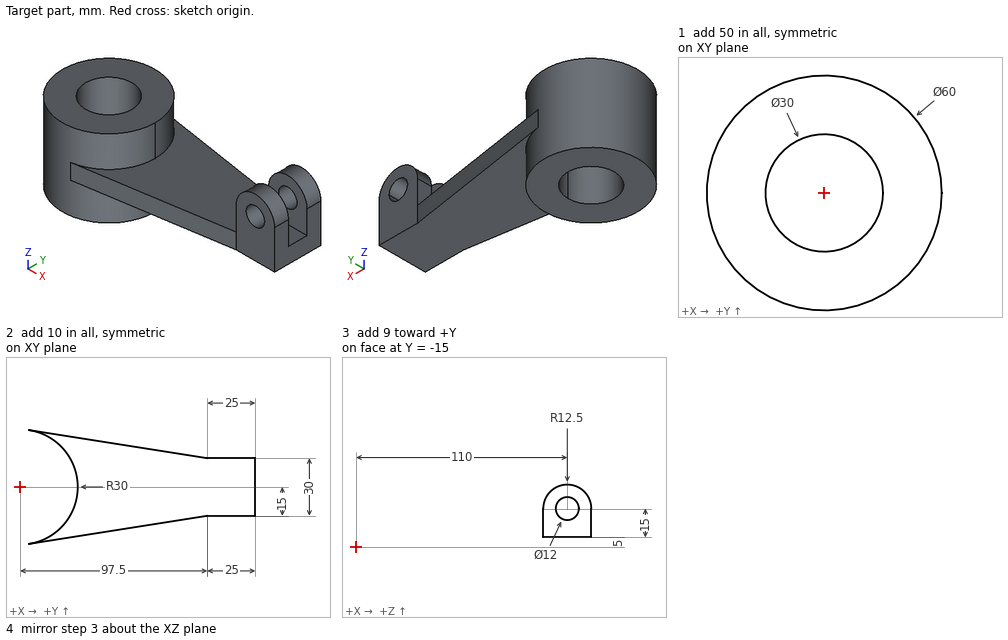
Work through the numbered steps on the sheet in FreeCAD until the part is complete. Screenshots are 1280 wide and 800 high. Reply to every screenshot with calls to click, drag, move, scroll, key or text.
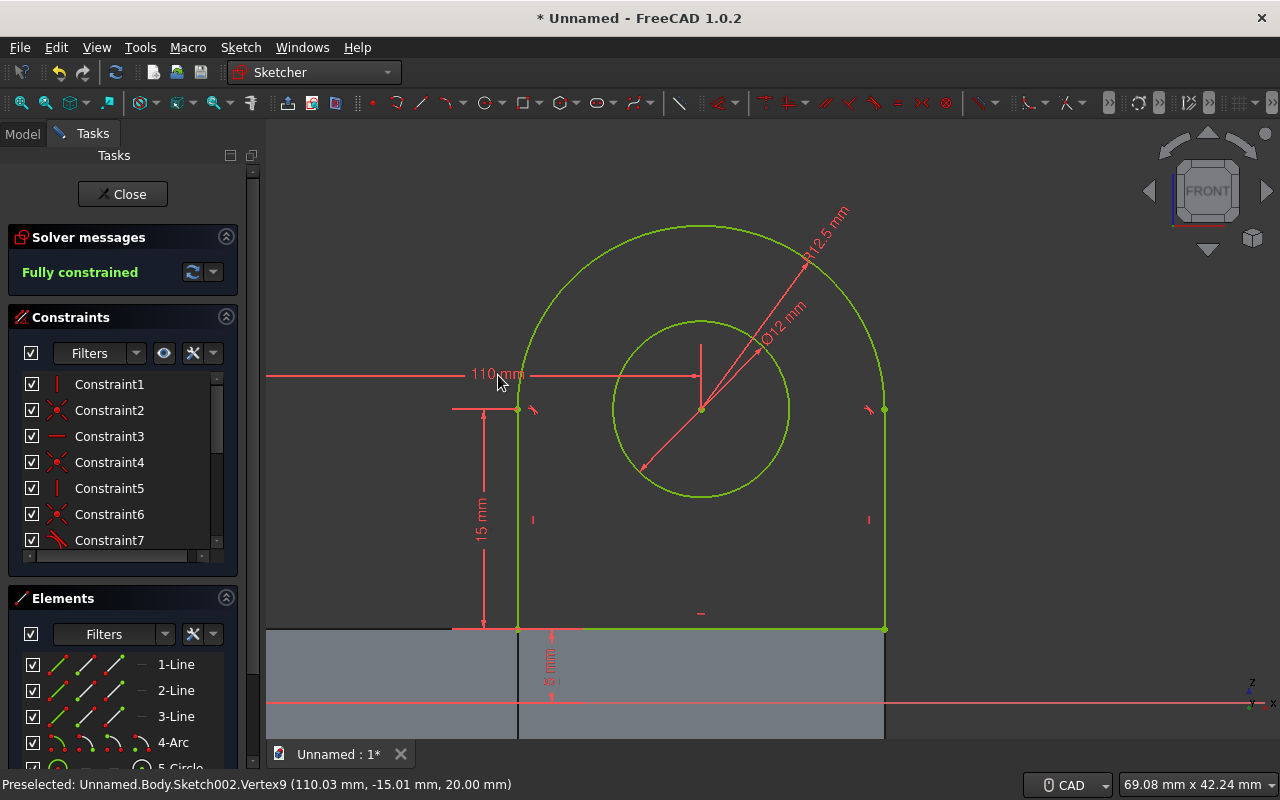
click(123, 194)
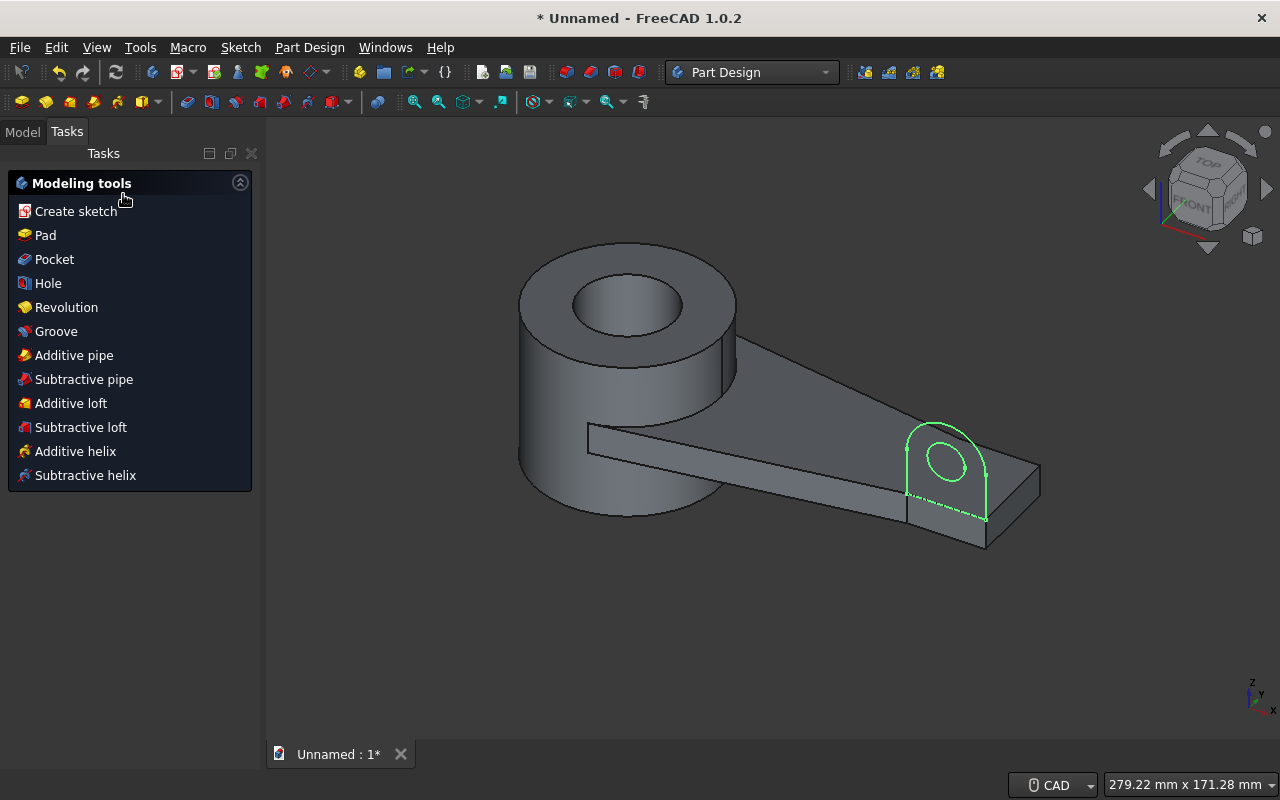
click(22, 102)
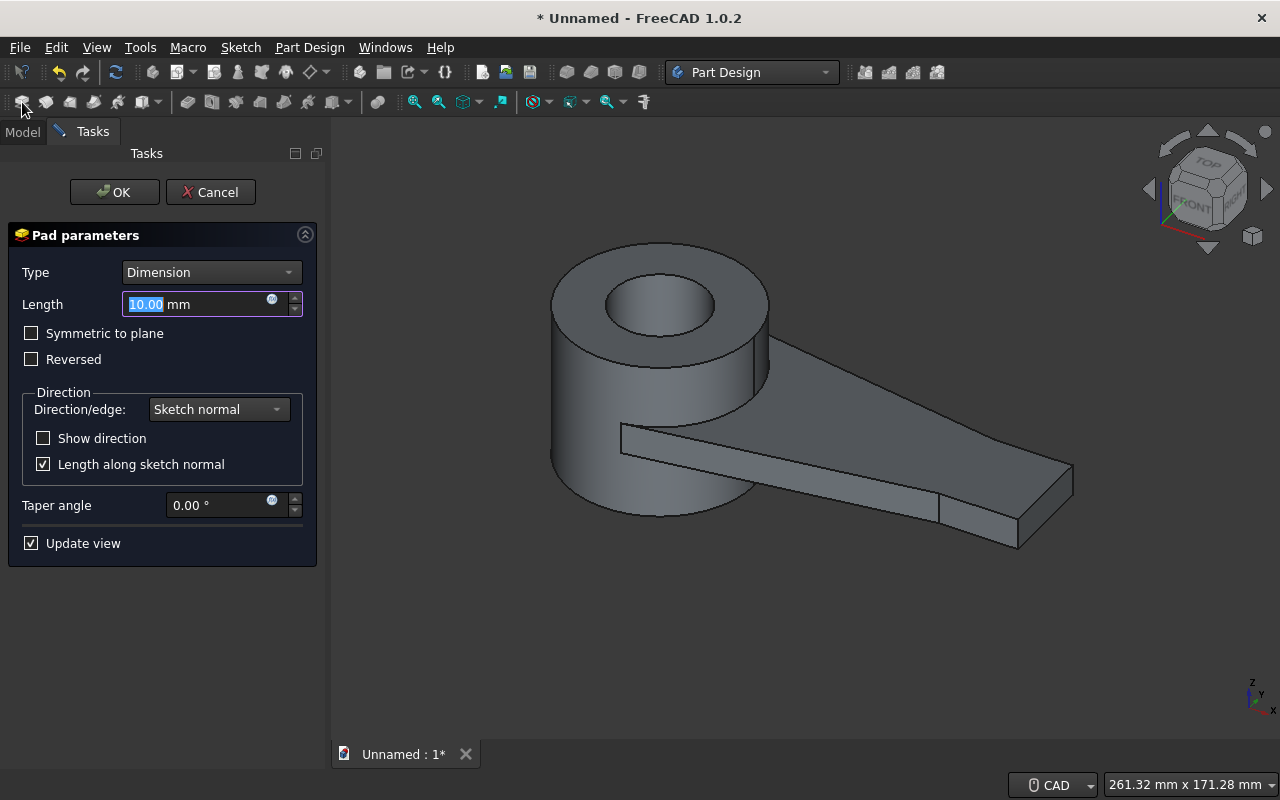
text(9)
key(Tab)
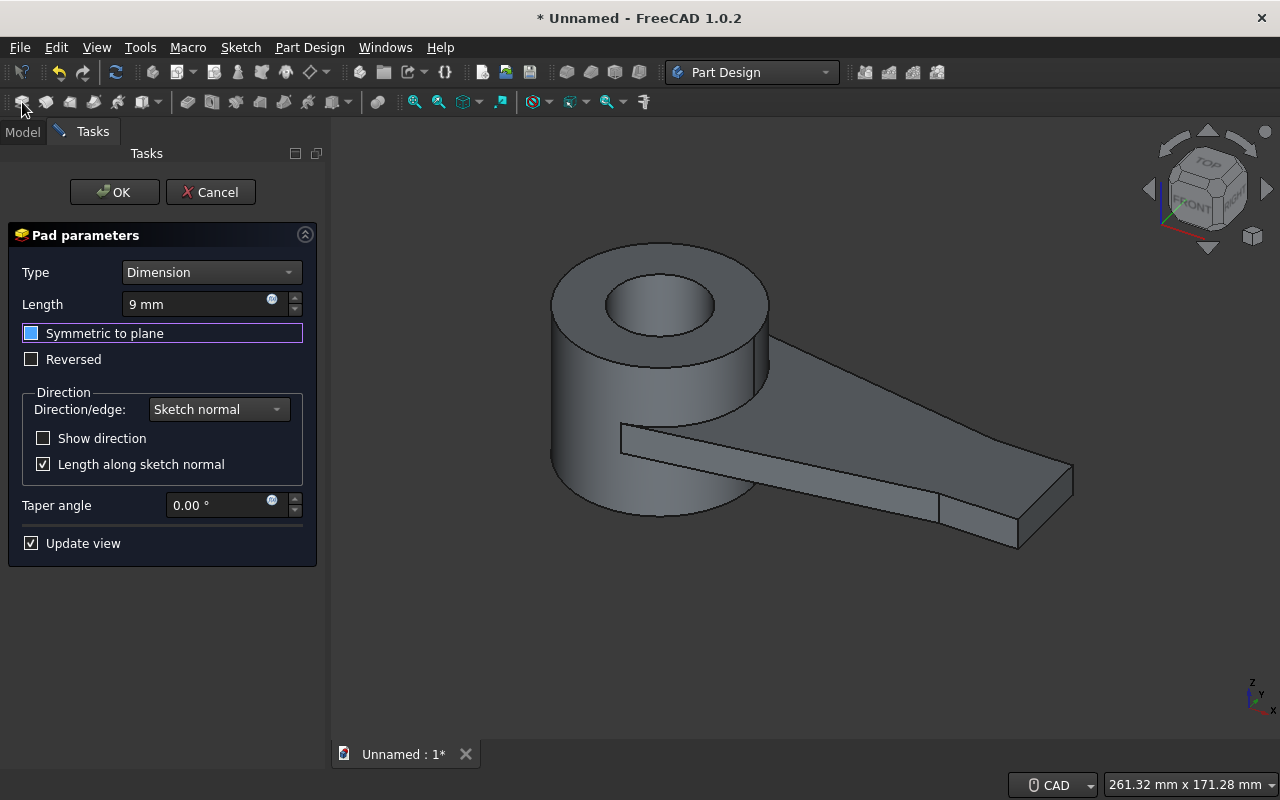
click(30, 359)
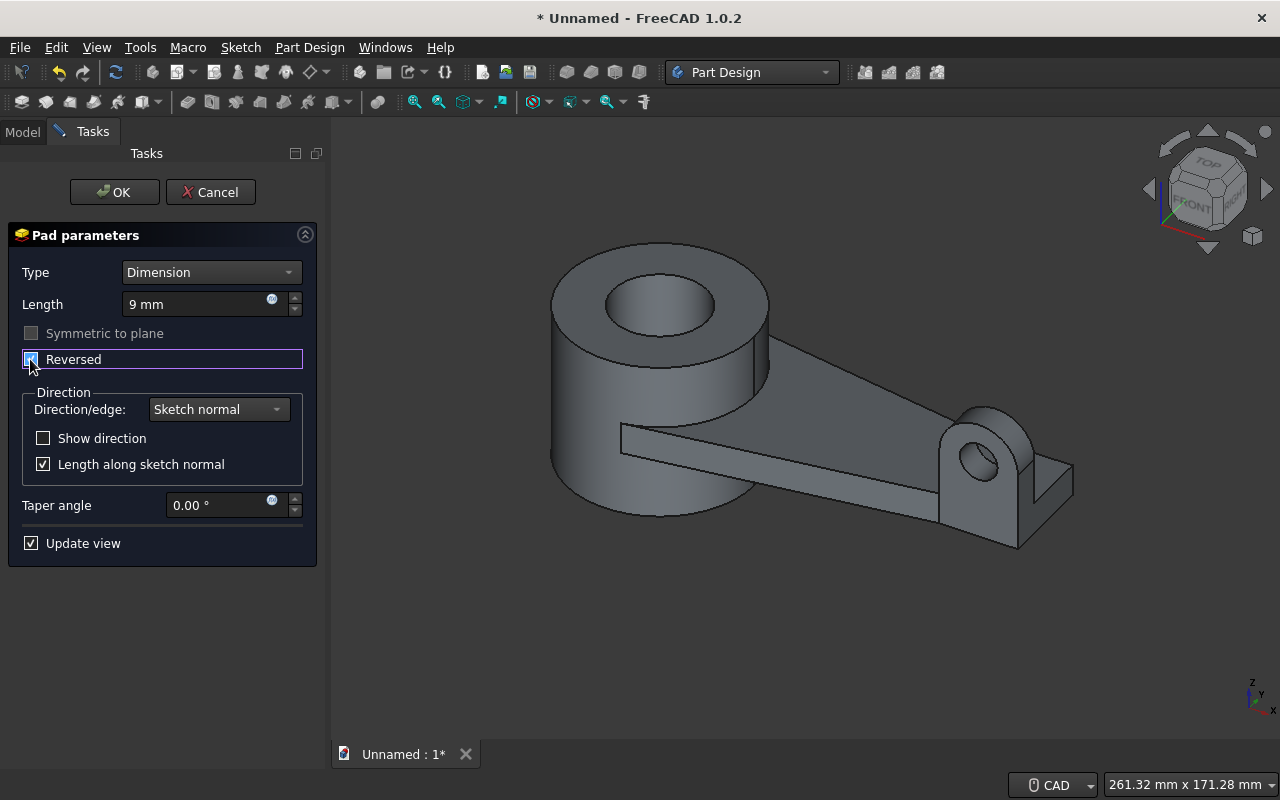
click(115, 192)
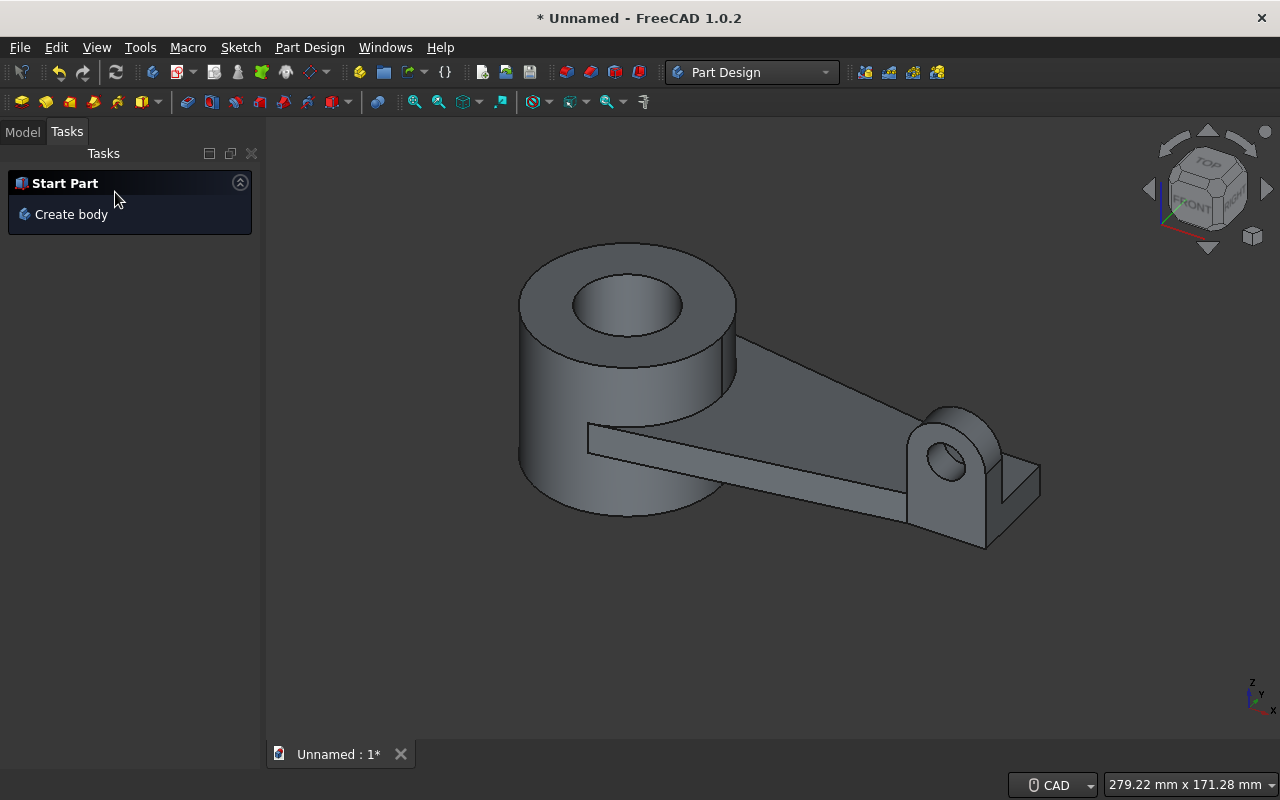
click(23, 131)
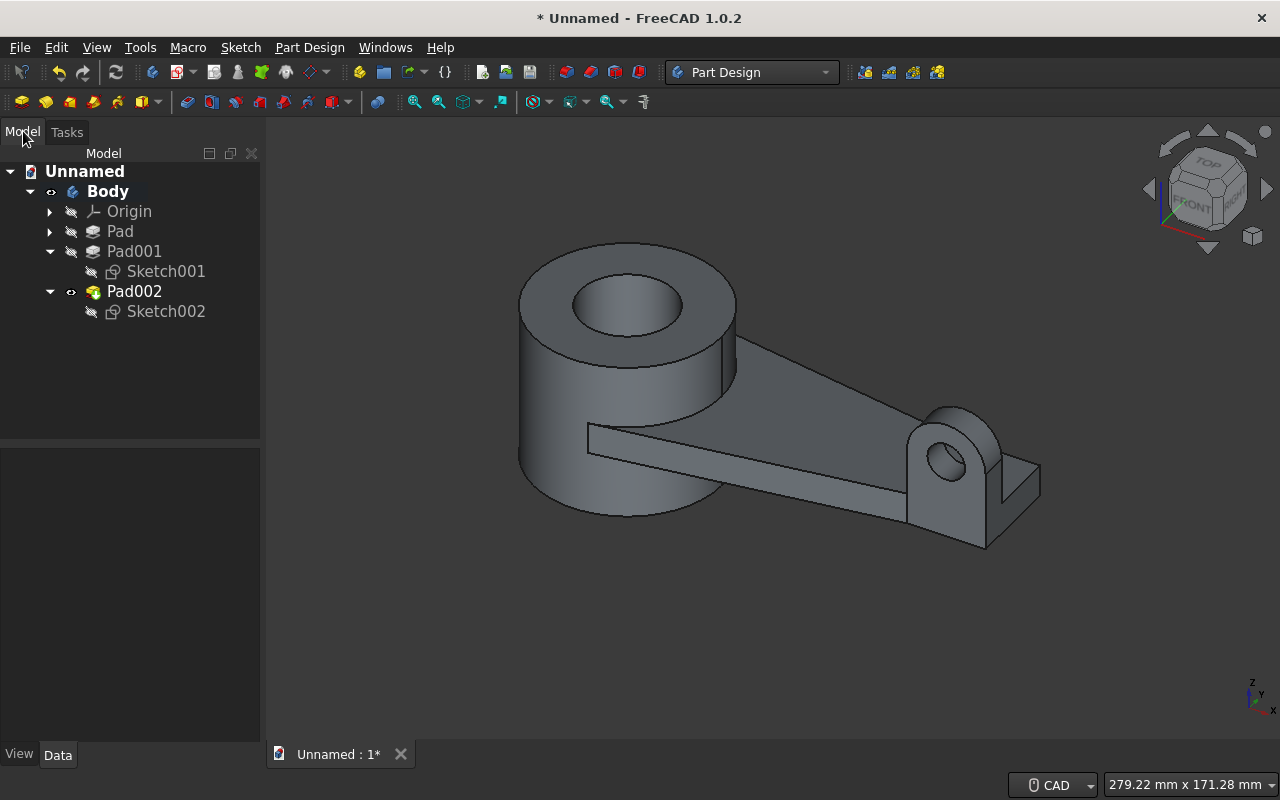
click(116, 292)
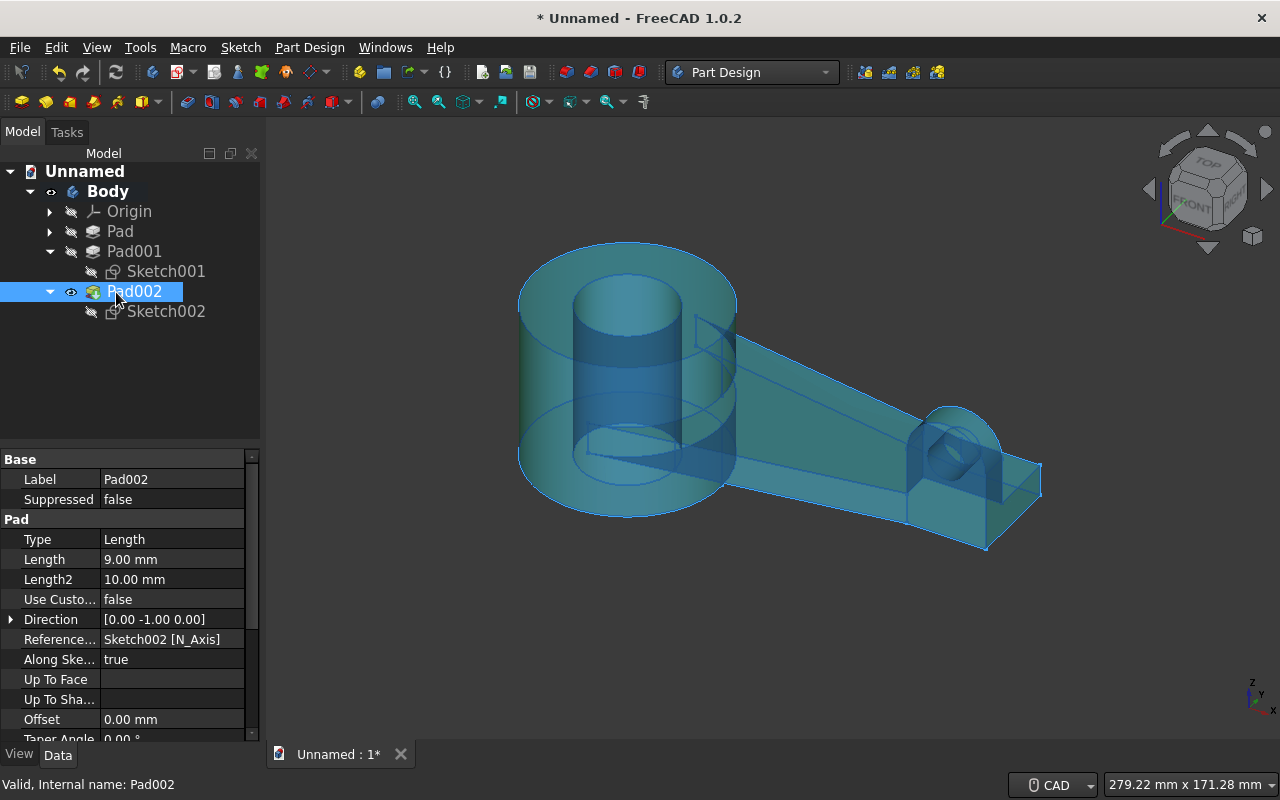
click(866, 72)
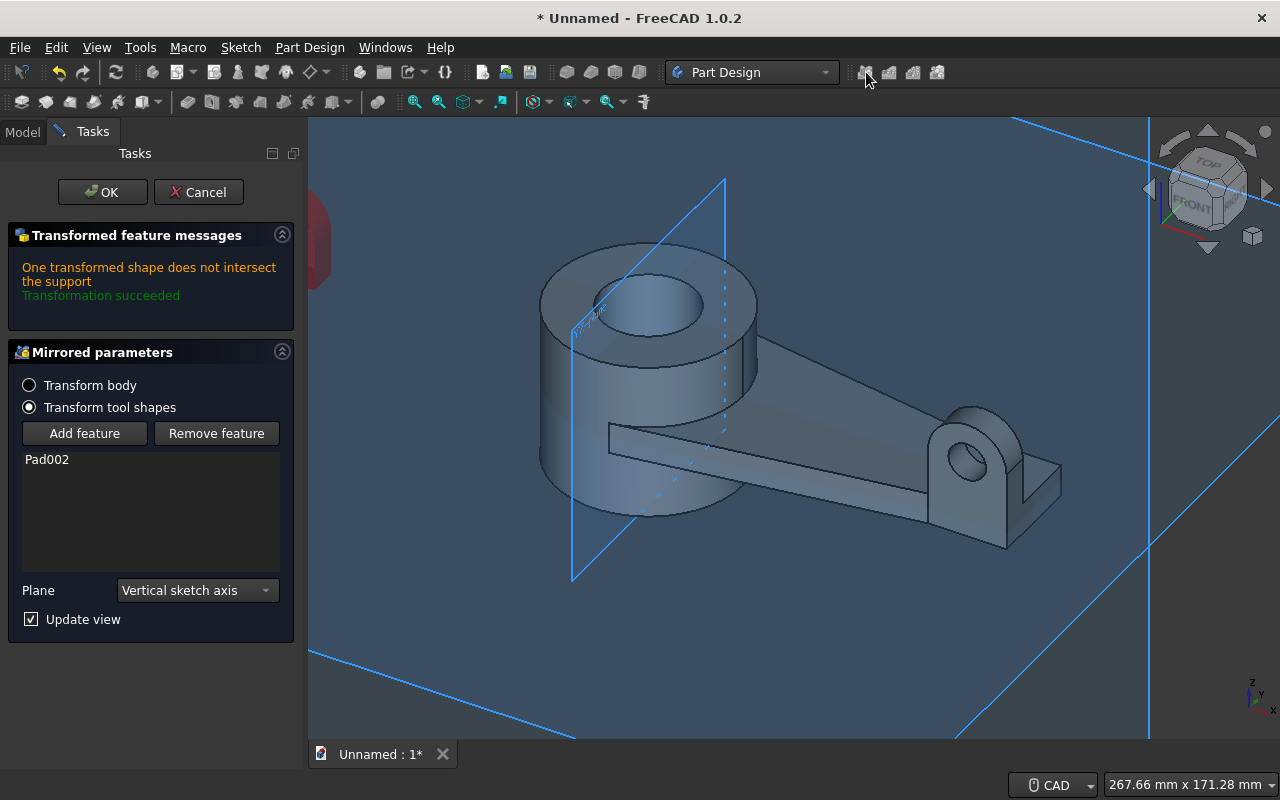
click(198, 590)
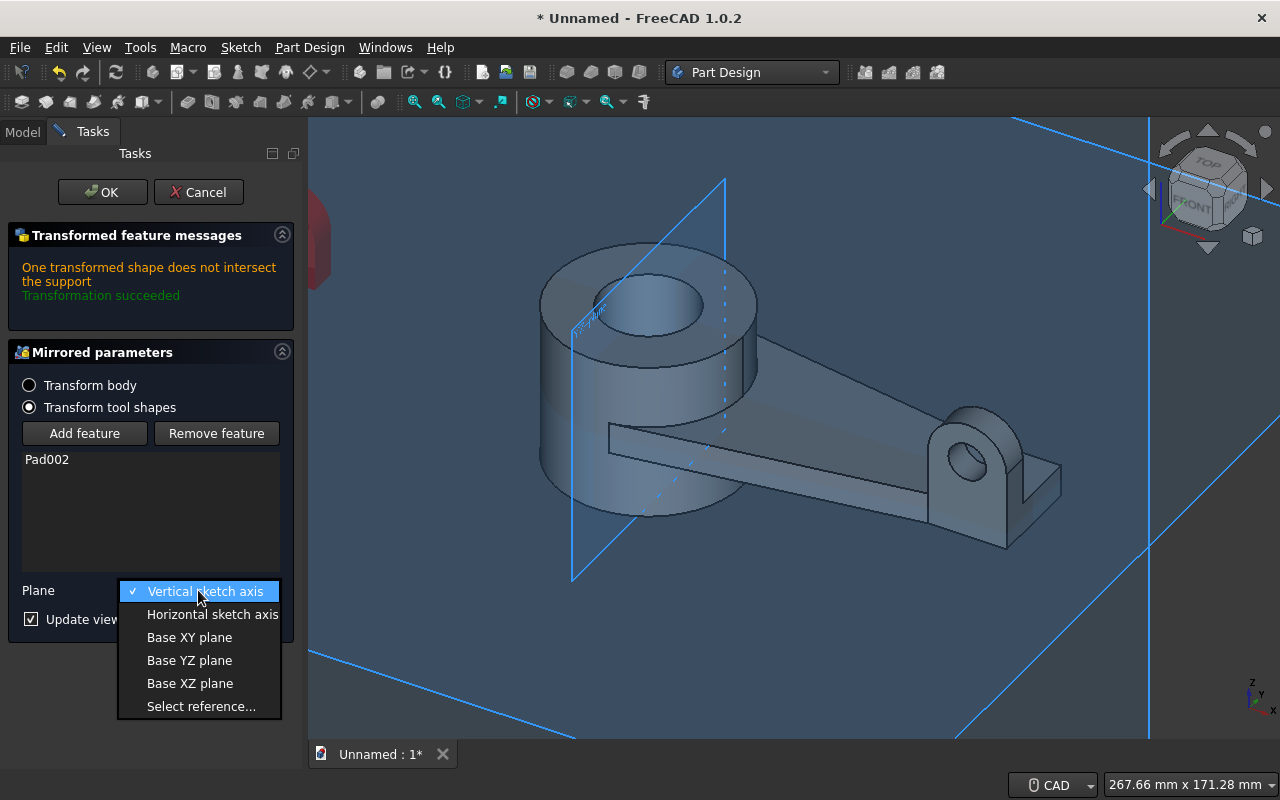
click(198, 684)